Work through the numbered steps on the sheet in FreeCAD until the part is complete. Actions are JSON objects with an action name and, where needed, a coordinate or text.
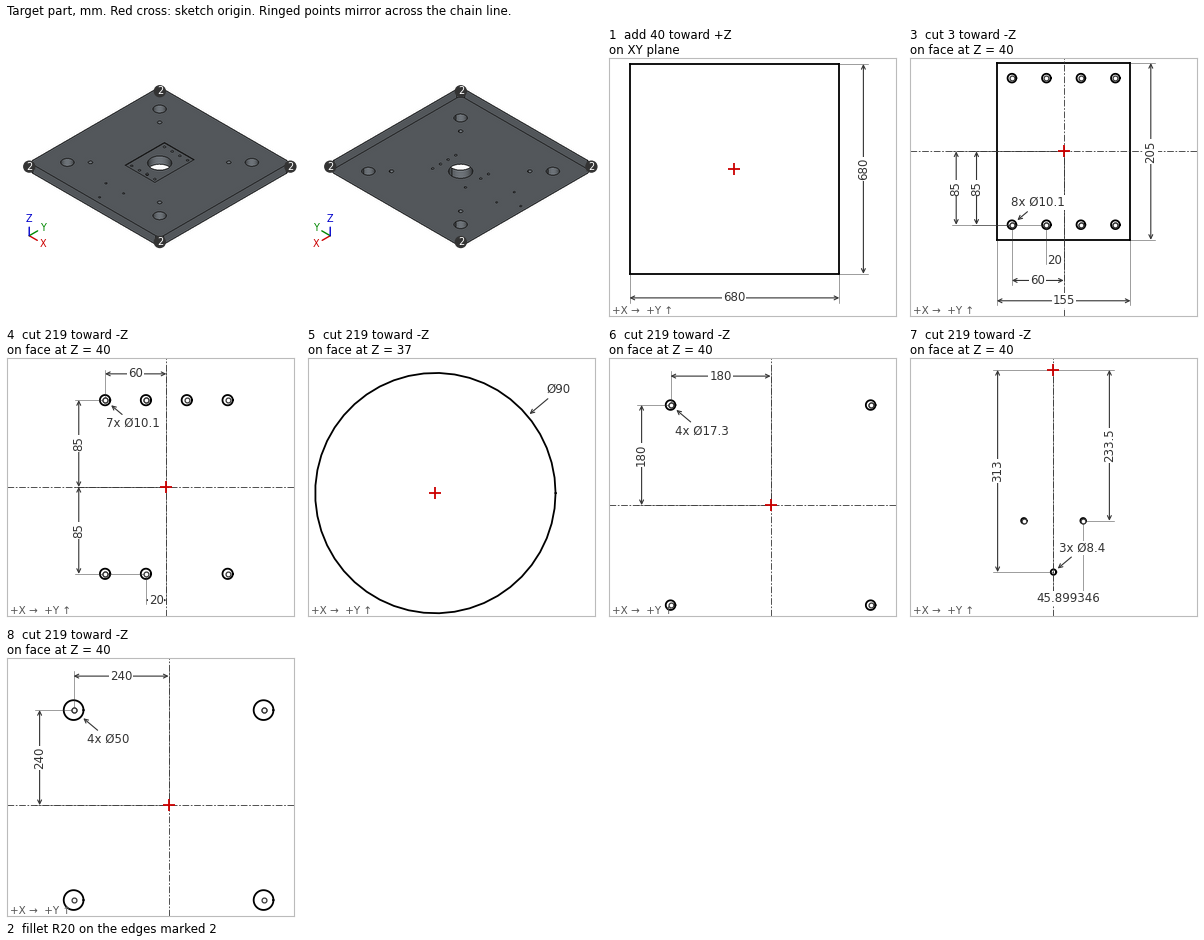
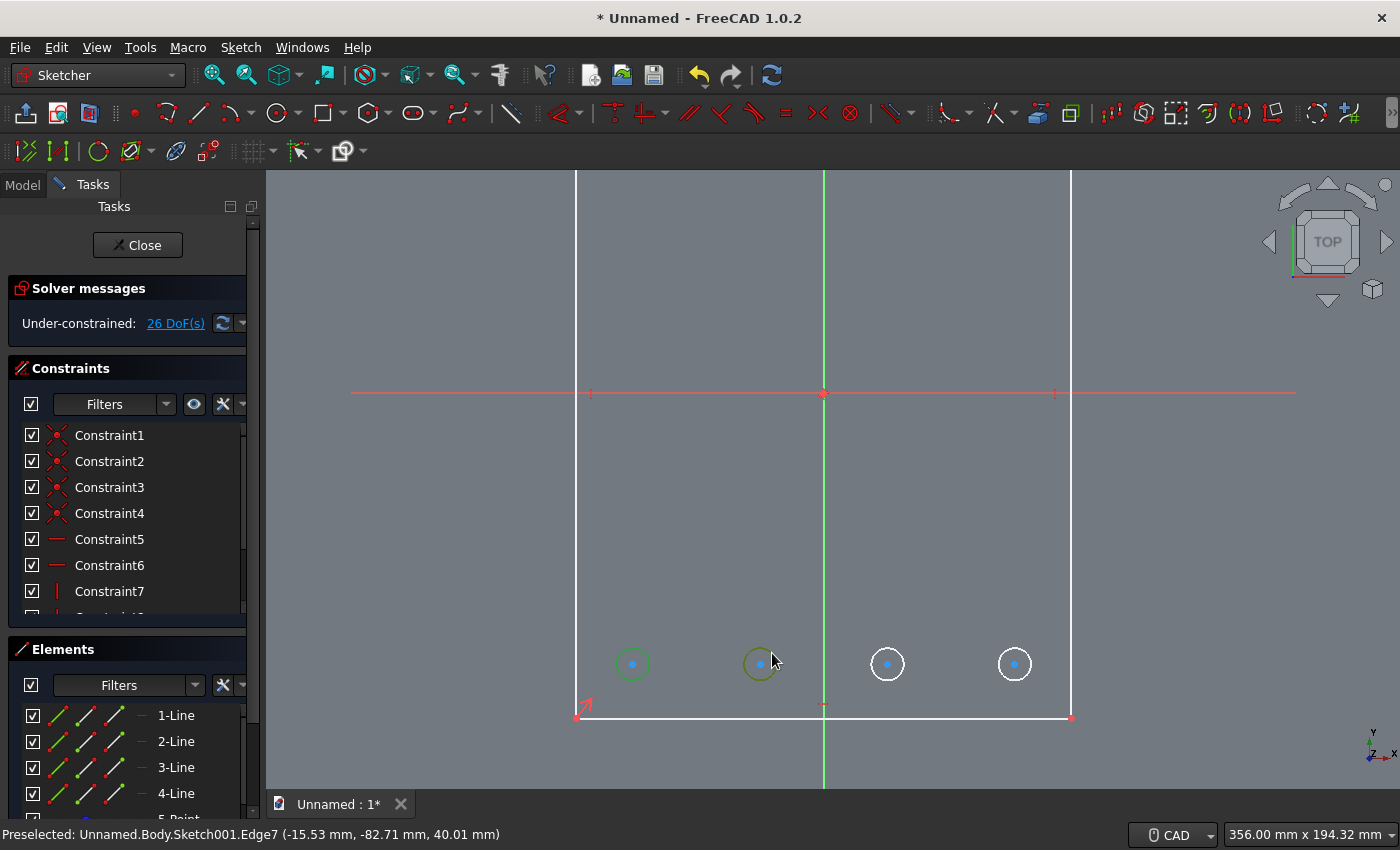
{"action": "left_click", "coordinate": [899, 653]}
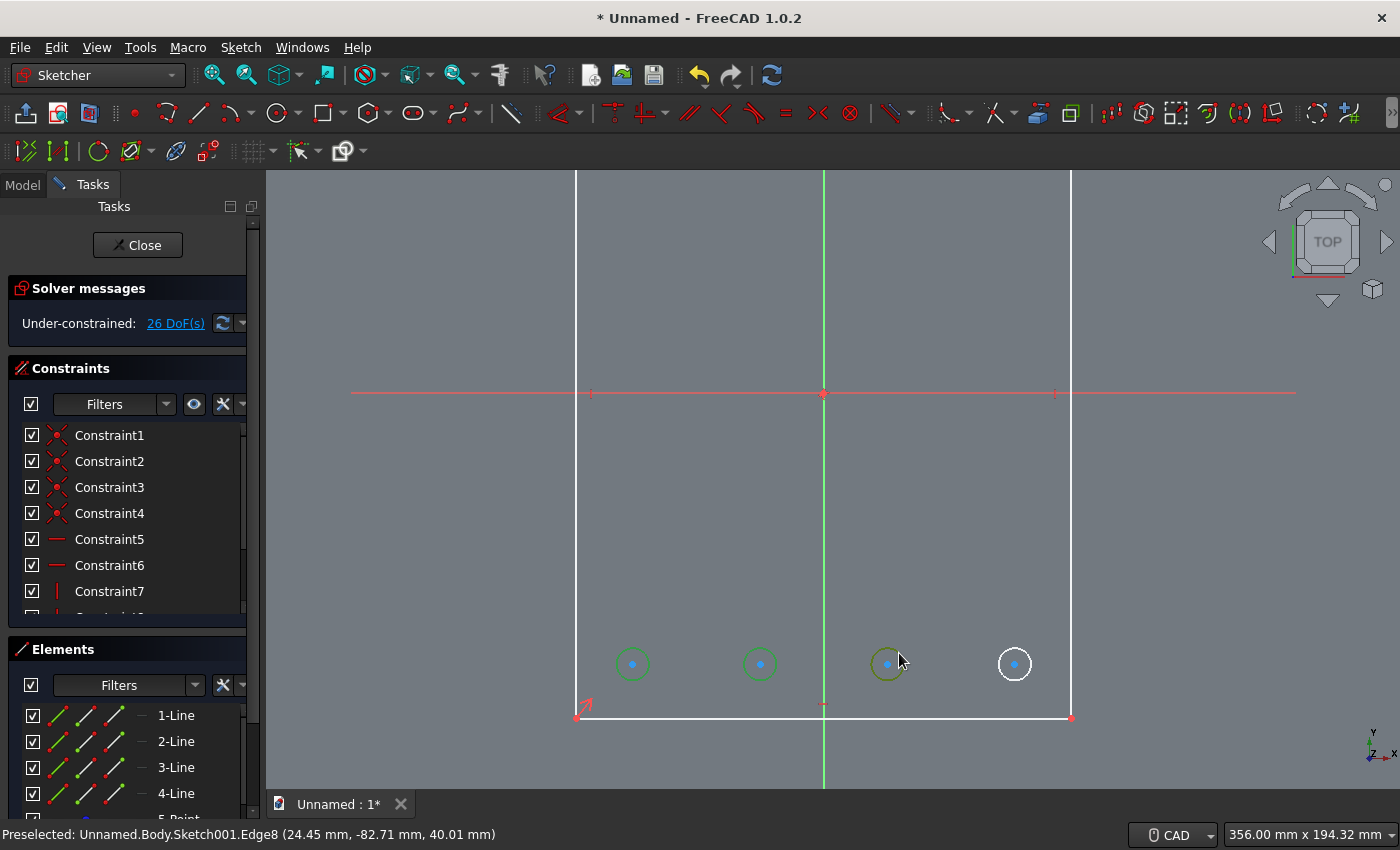
{"action": "left_click", "coordinate": [1026, 653]}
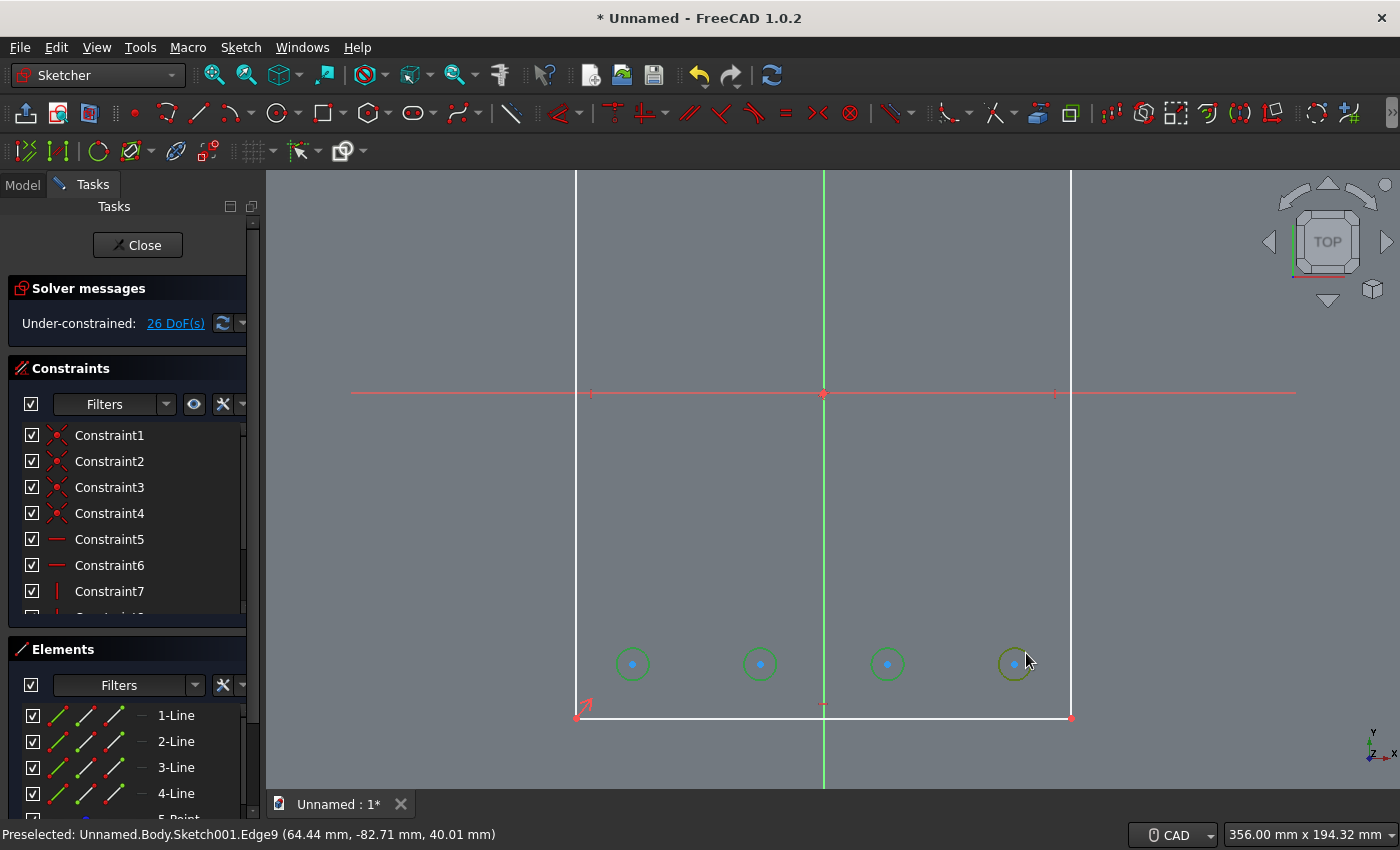
{"action": "scroll", "coordinate": [644, 655], "scroll_direction": "down", "scroll_amount": 2}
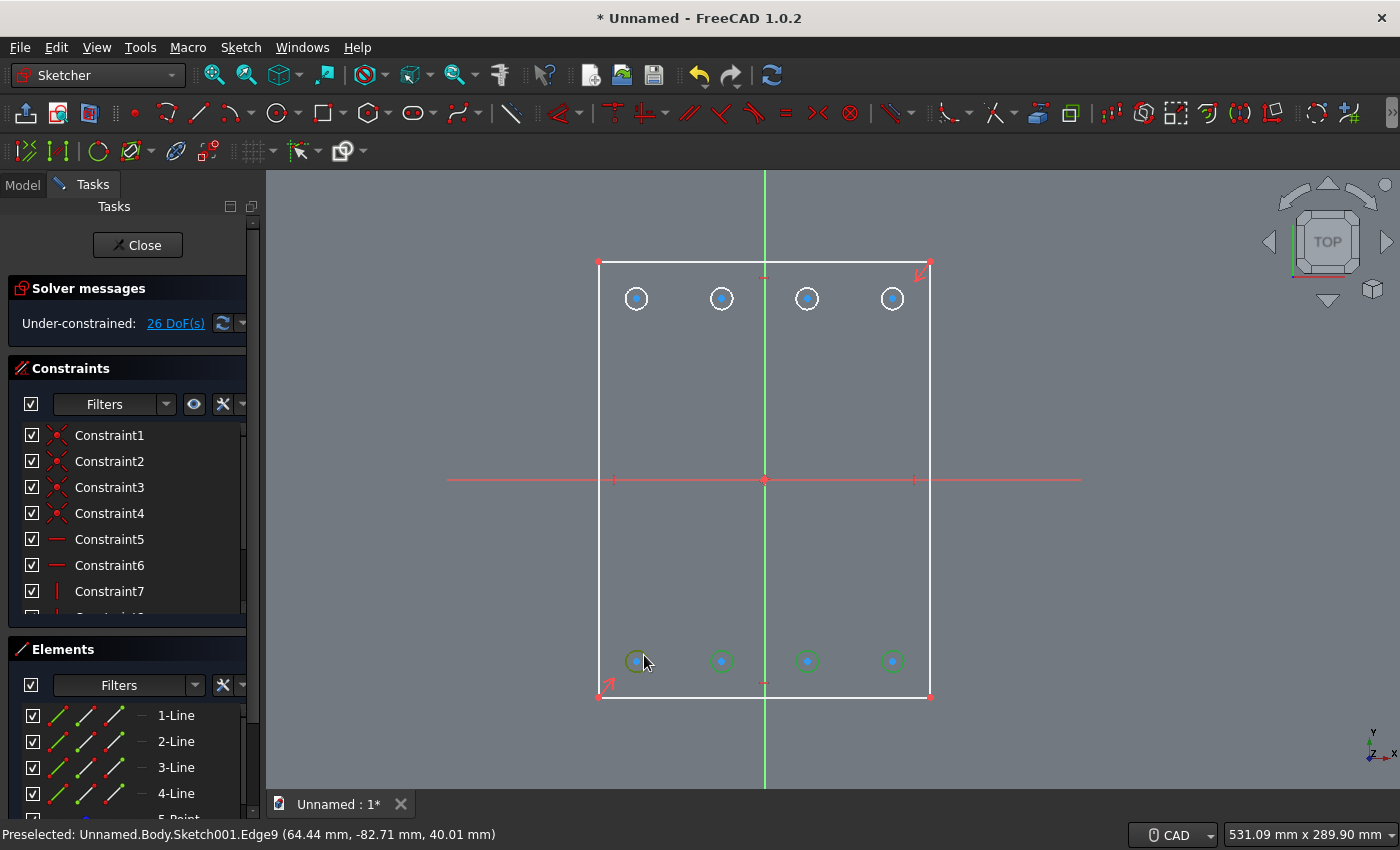
{"action": "scroll", "coordinate": [644, 291], "scroll_direction": "up", "scroll_amount": 2}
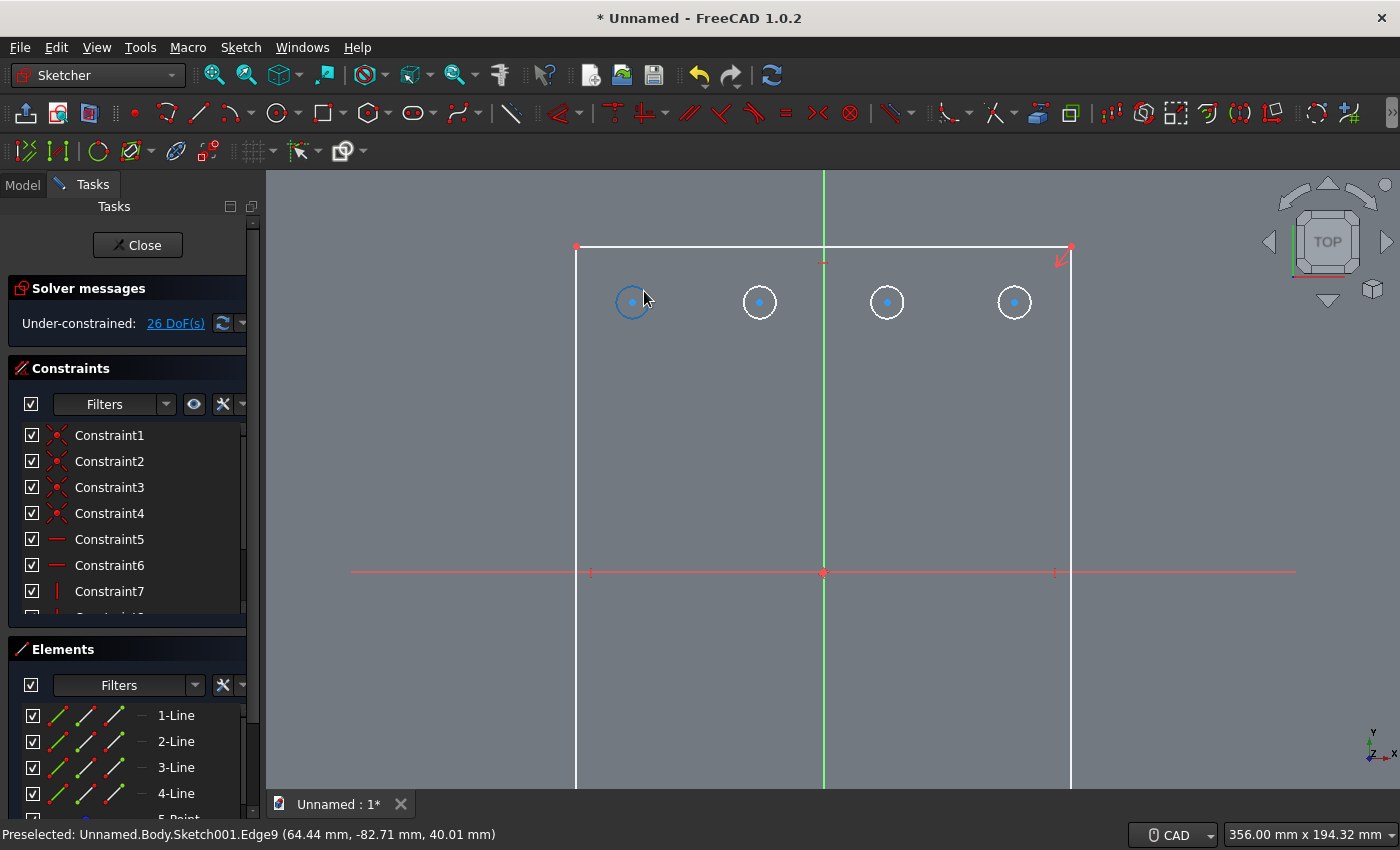
{"action": "left_click", "coordinate": [644, 291]}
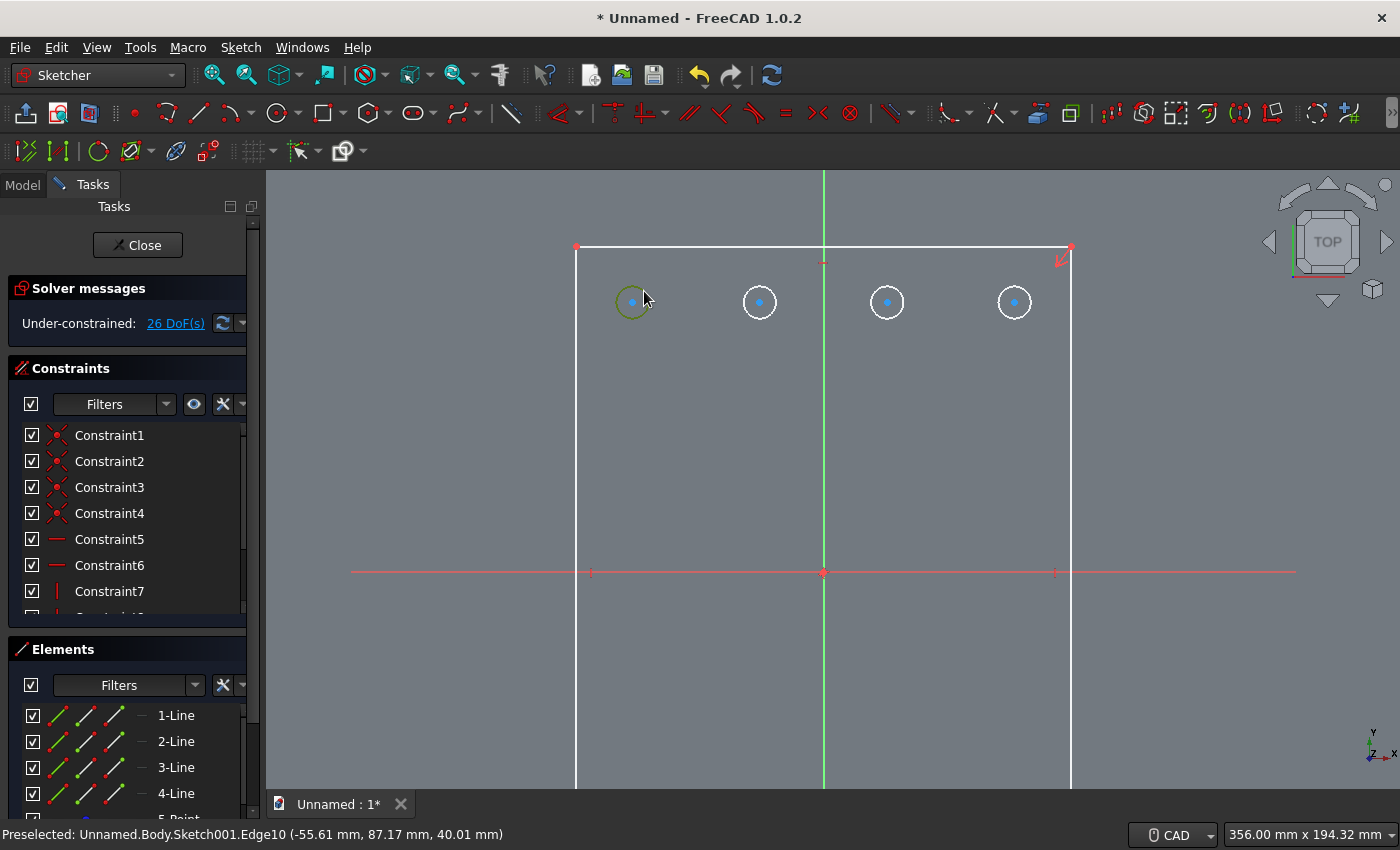
{"action": "left_click", "coordinate": [771, 291]}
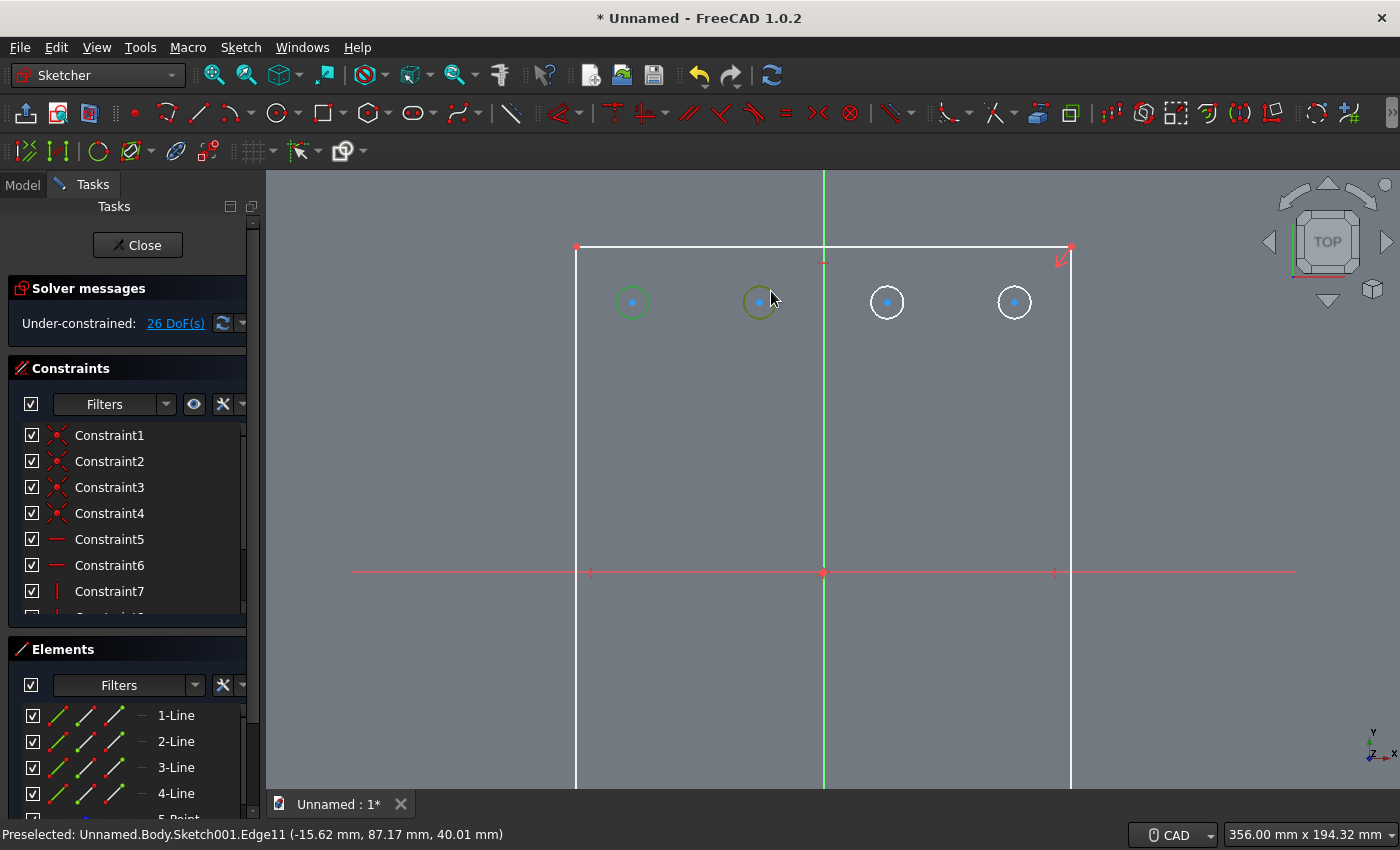
{"action": "left_click", "coordinate": [899, 291]}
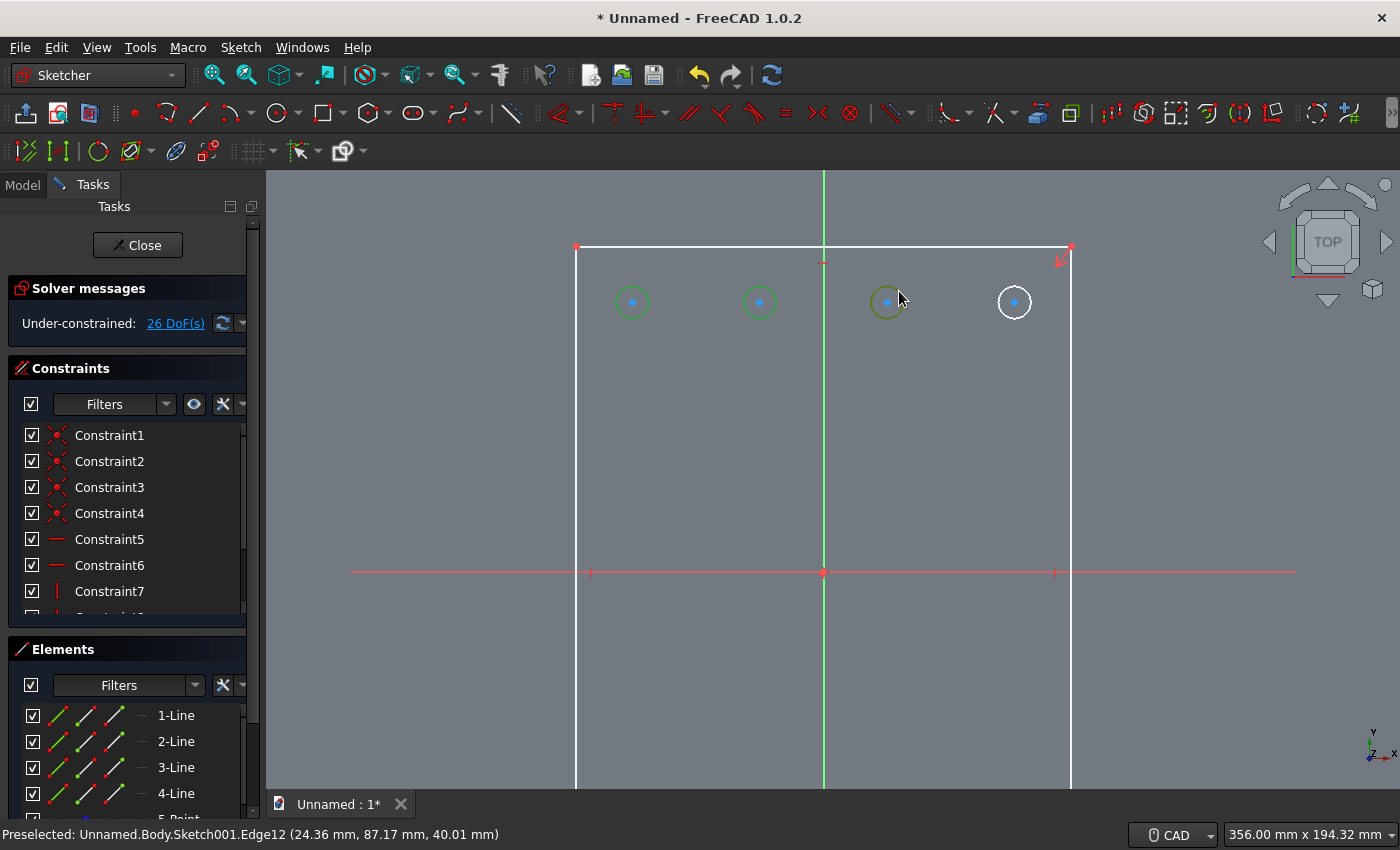
{"action": "left_click", "coordinate": [1026, 291]}